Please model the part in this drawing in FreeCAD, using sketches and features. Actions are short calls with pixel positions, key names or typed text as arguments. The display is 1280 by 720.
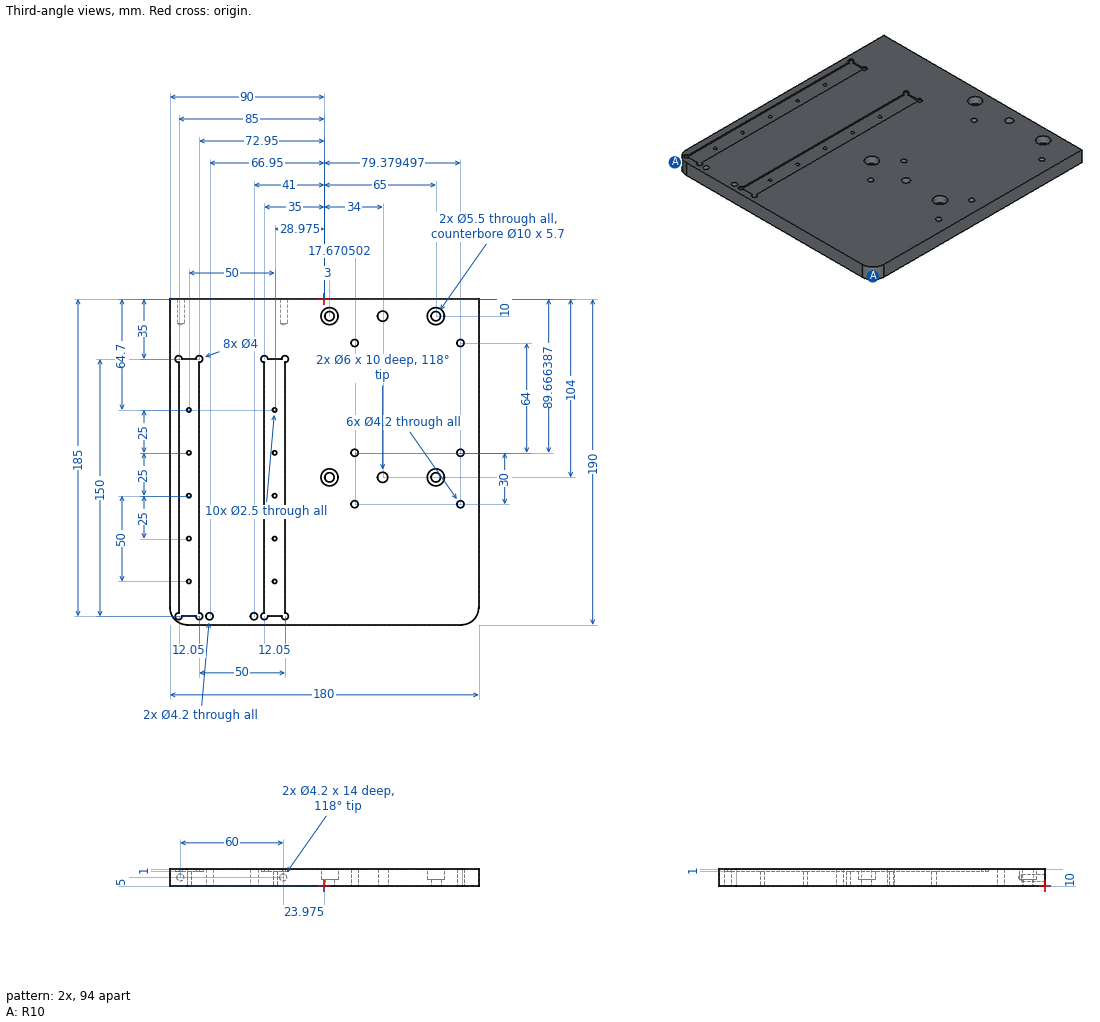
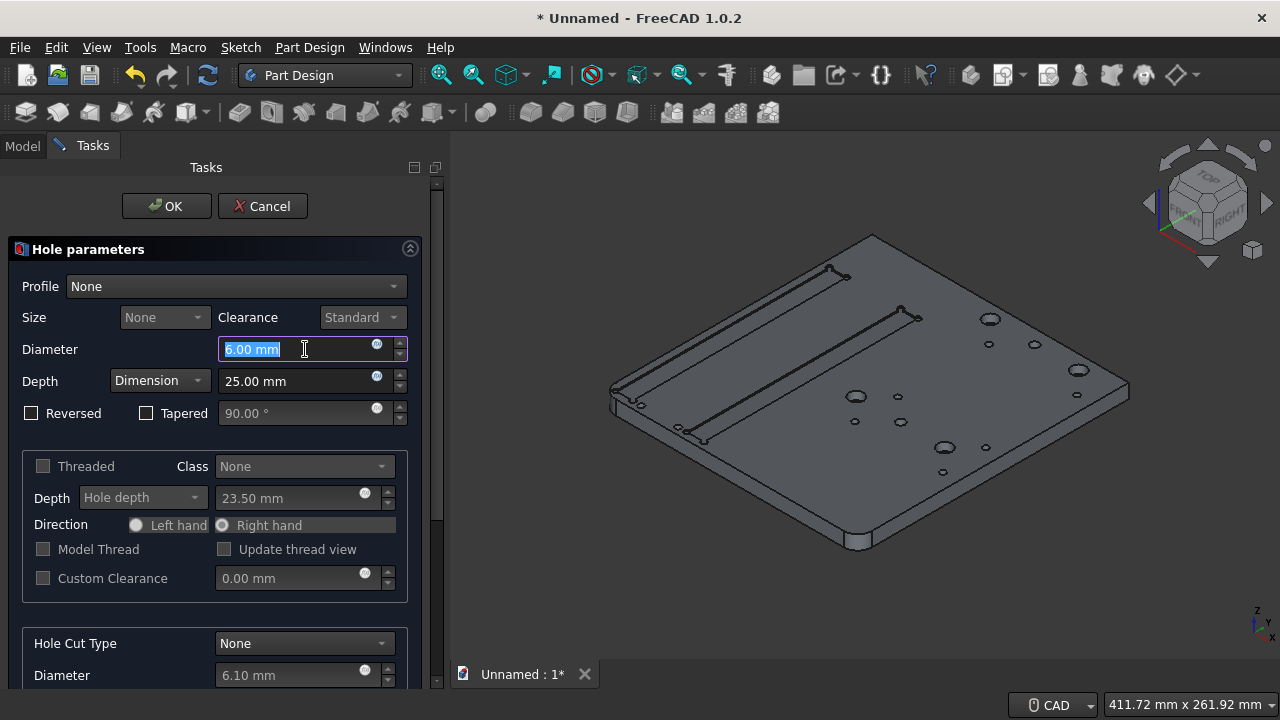
text(6)
key(Tab)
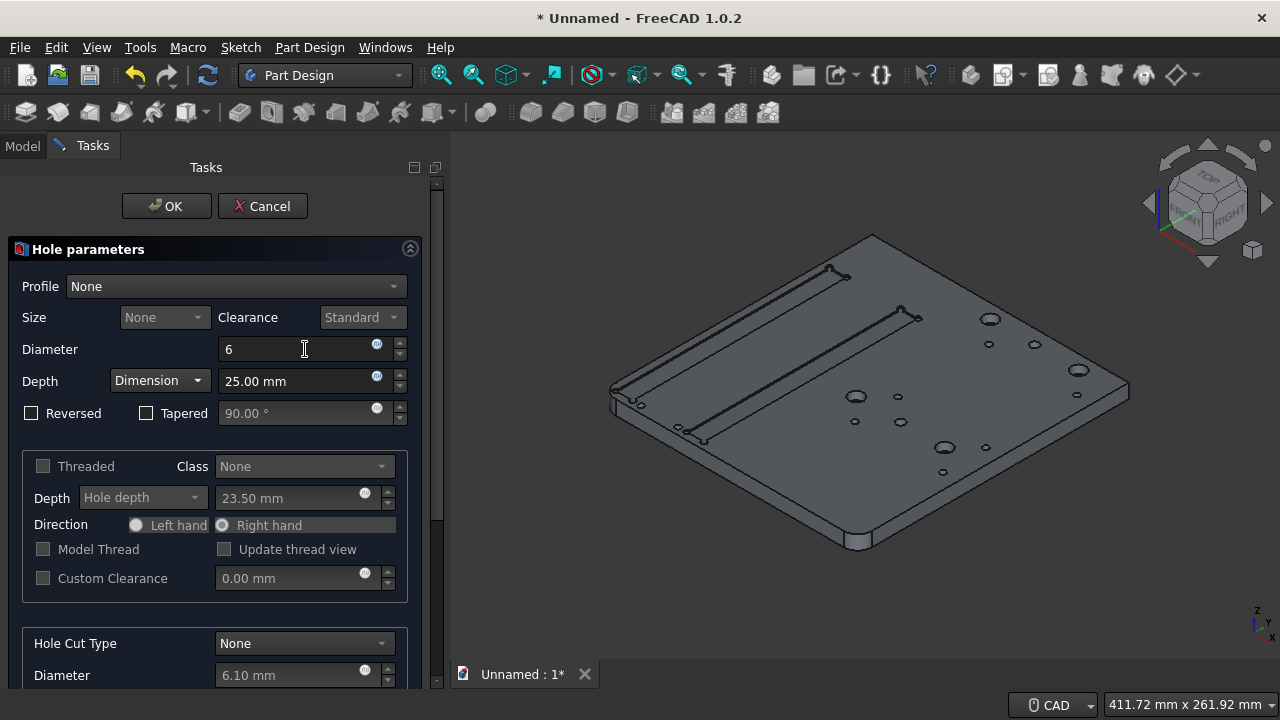
triple_click(305, 381)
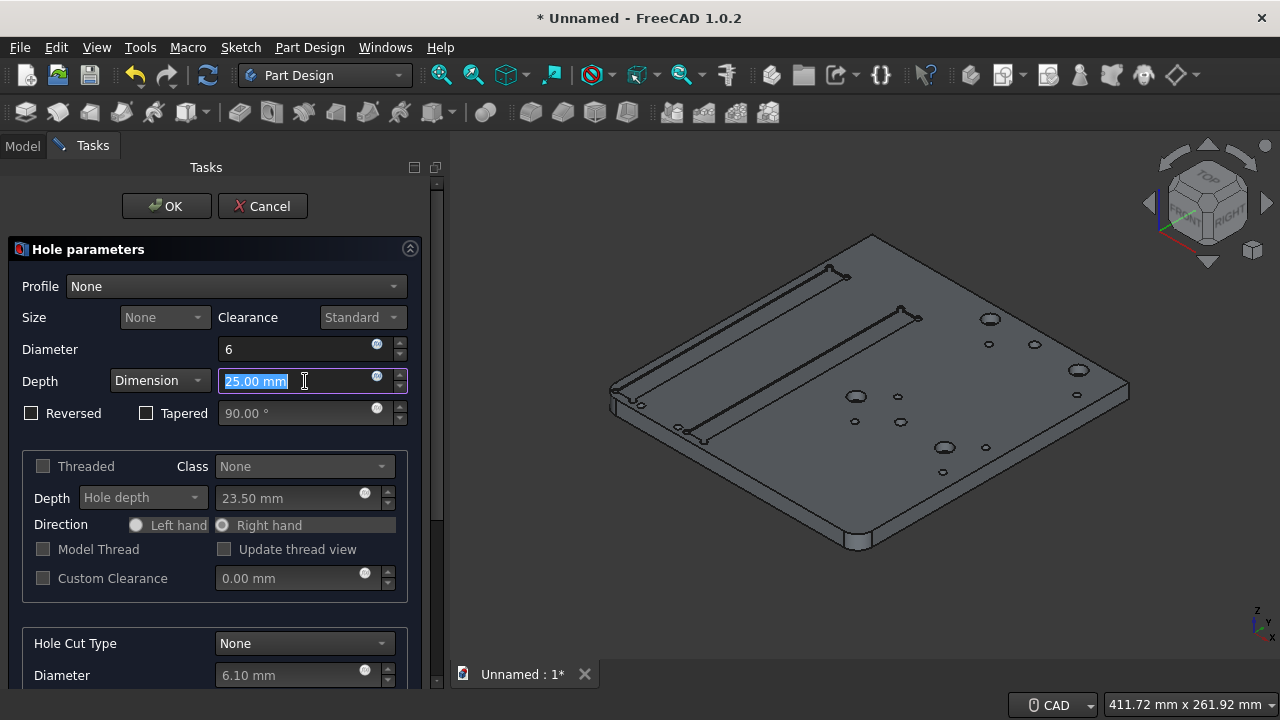
text(10)
key(Tab)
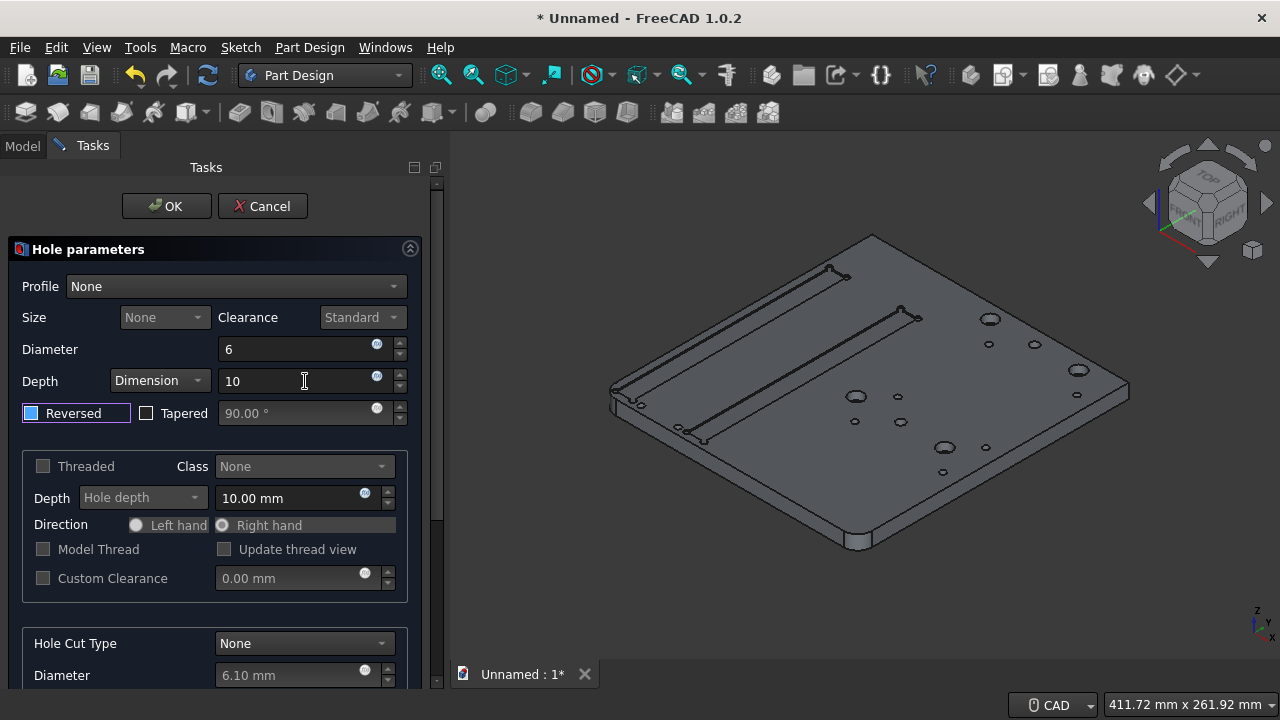
click(167, 206)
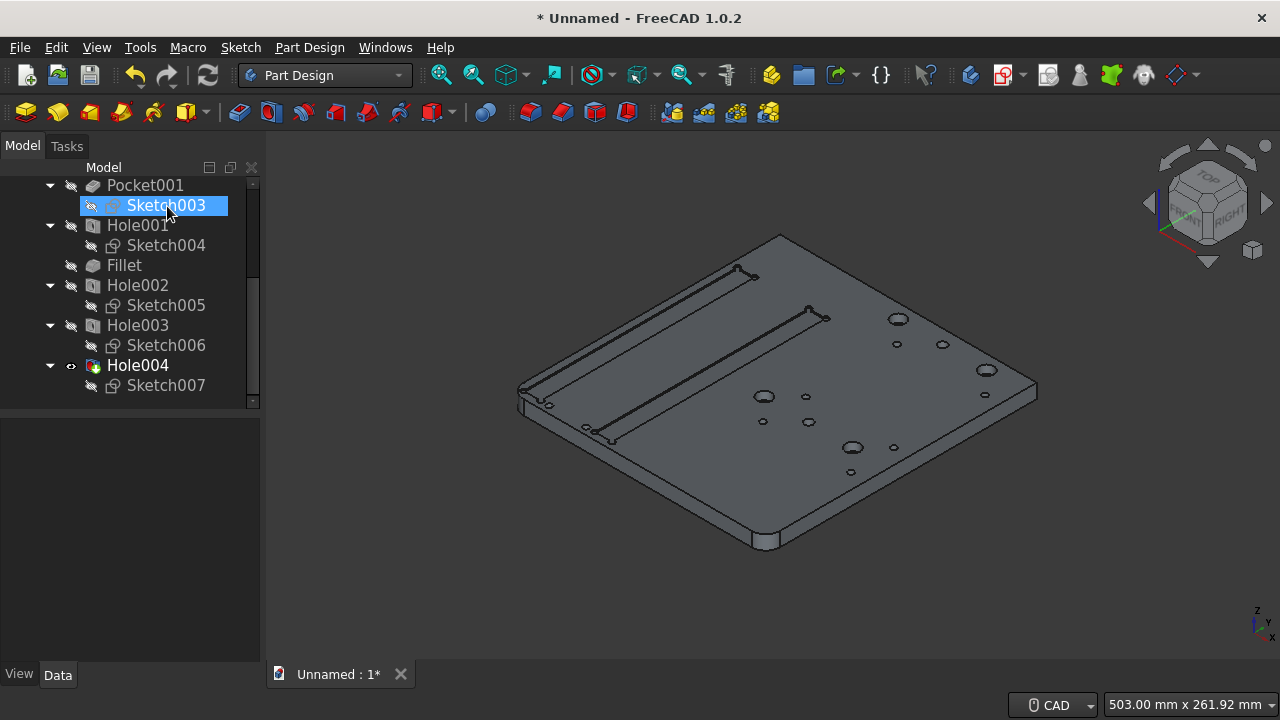
click(769, 473)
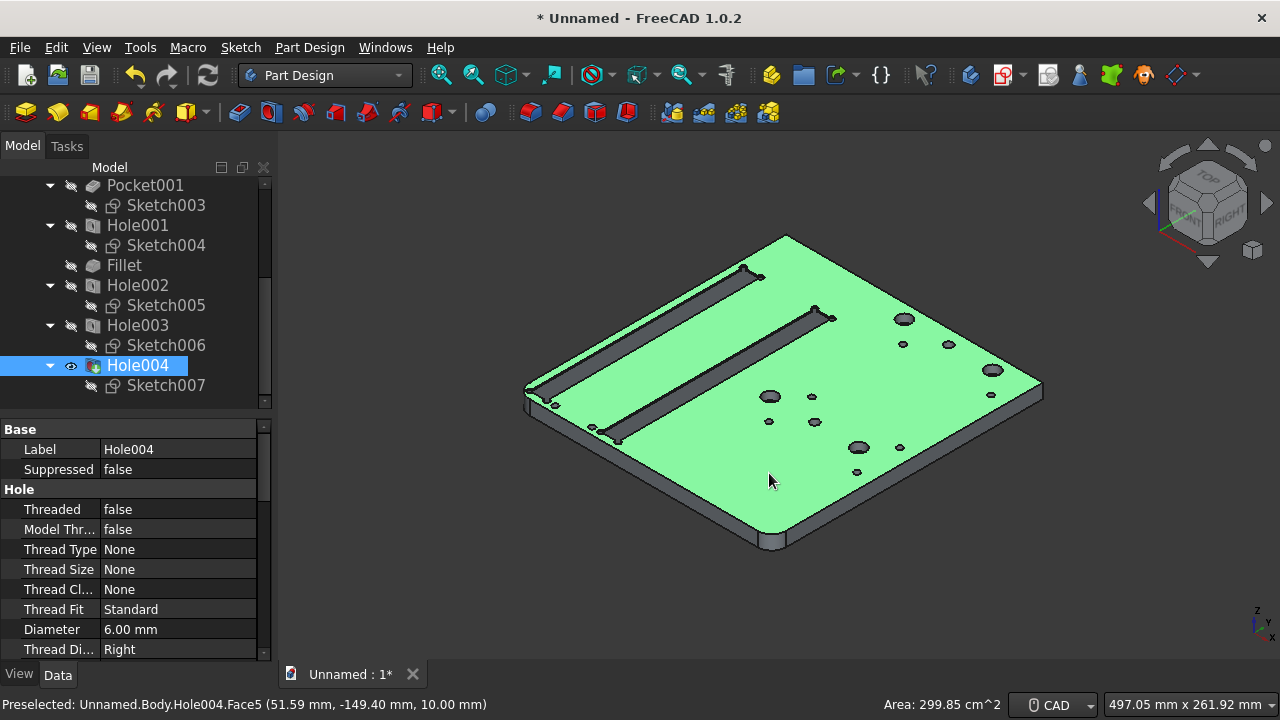
click(1004, 76)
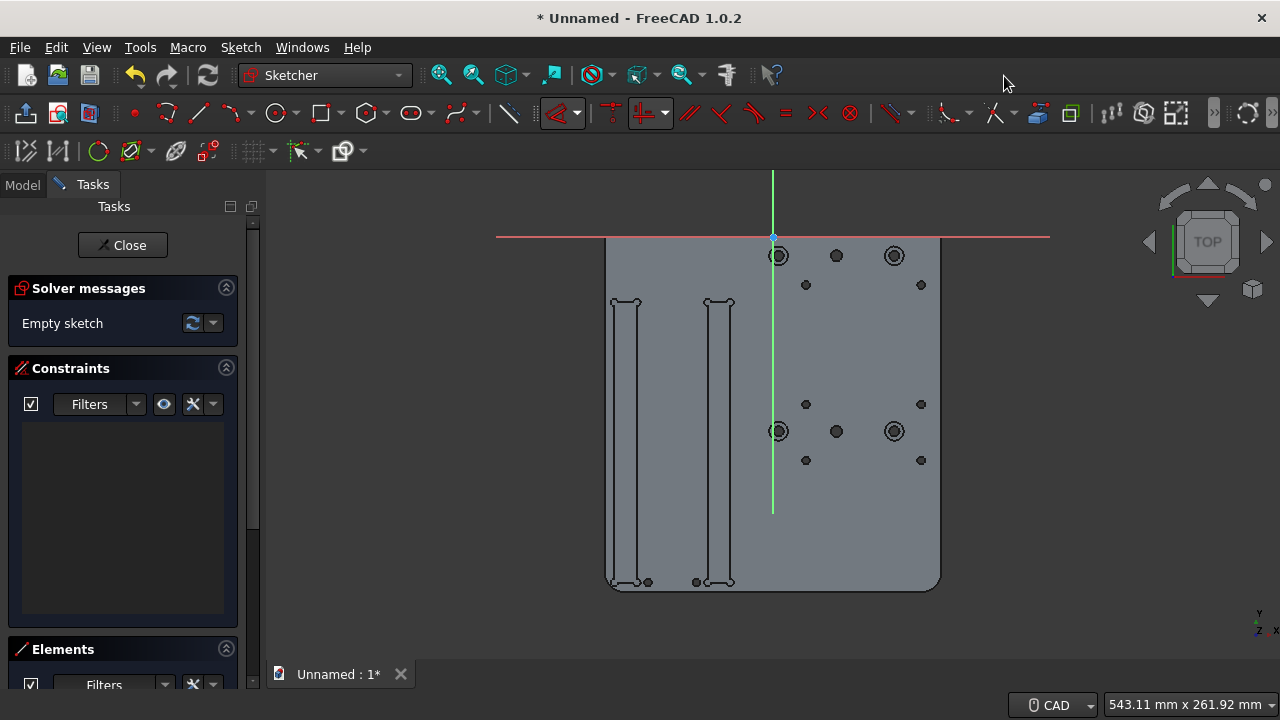
key(g)
key(c)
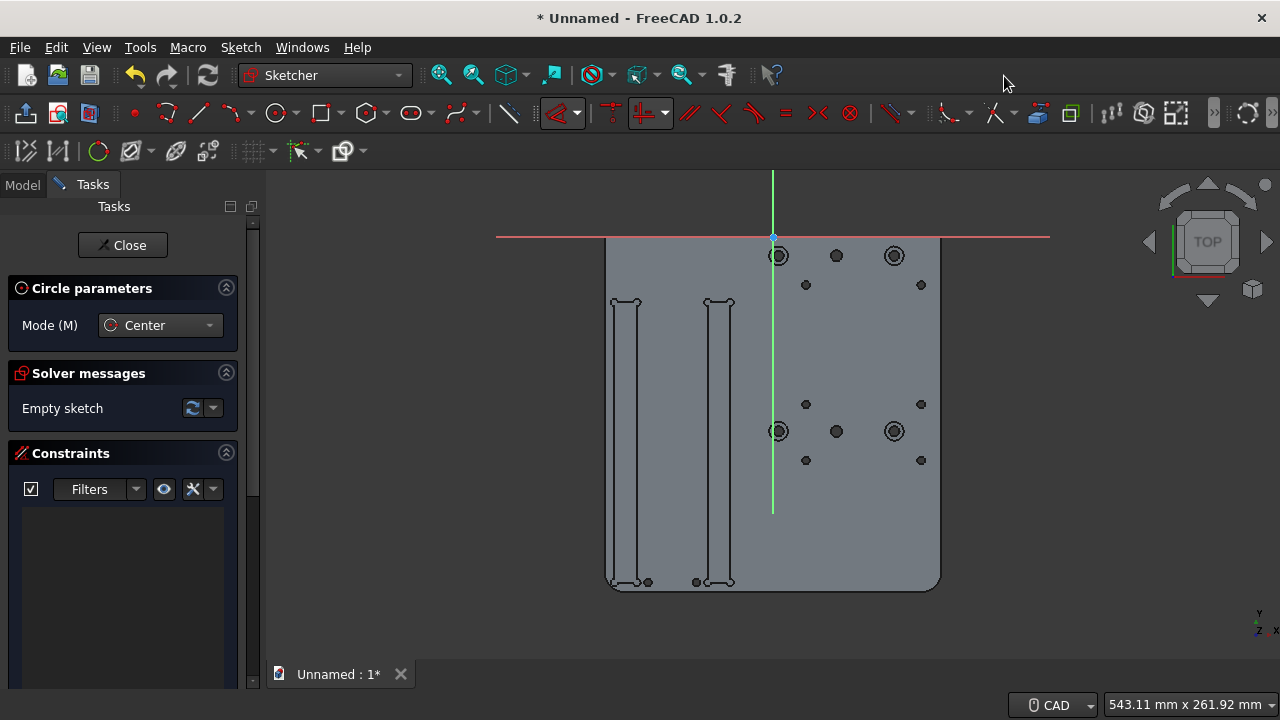
scroll(719, 358, up, 12)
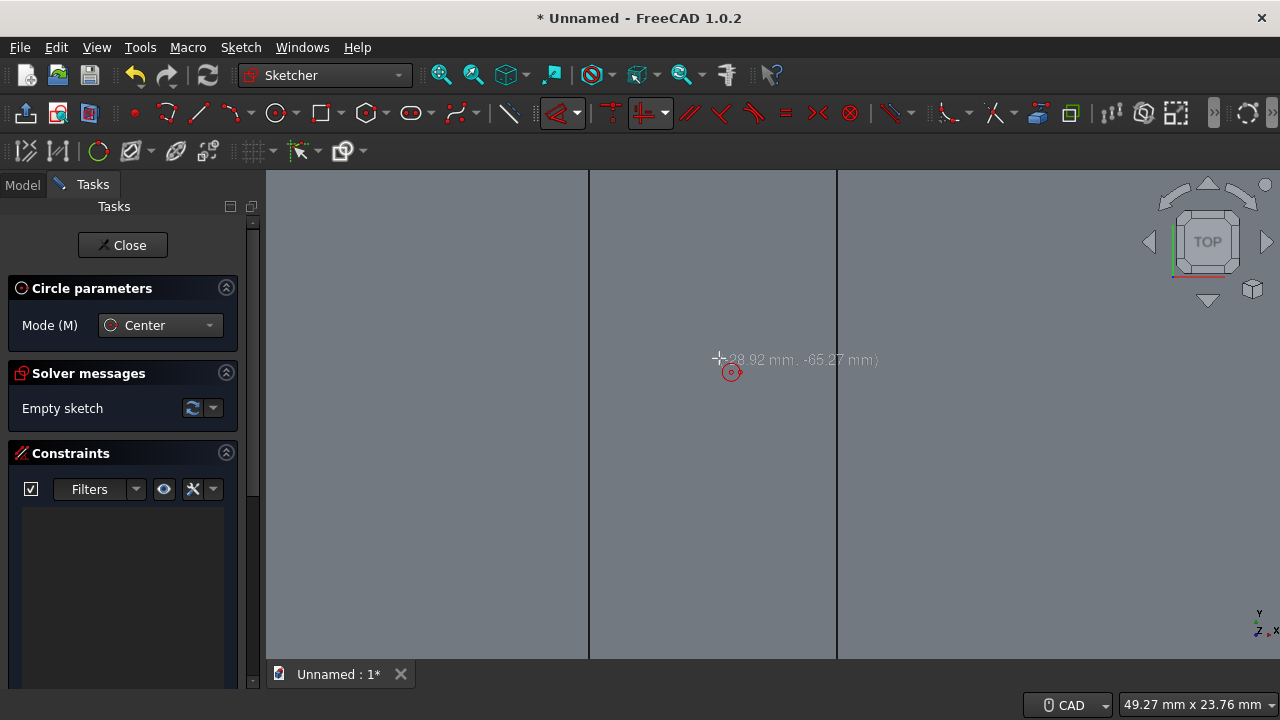
scroll(726, 383, down, 12)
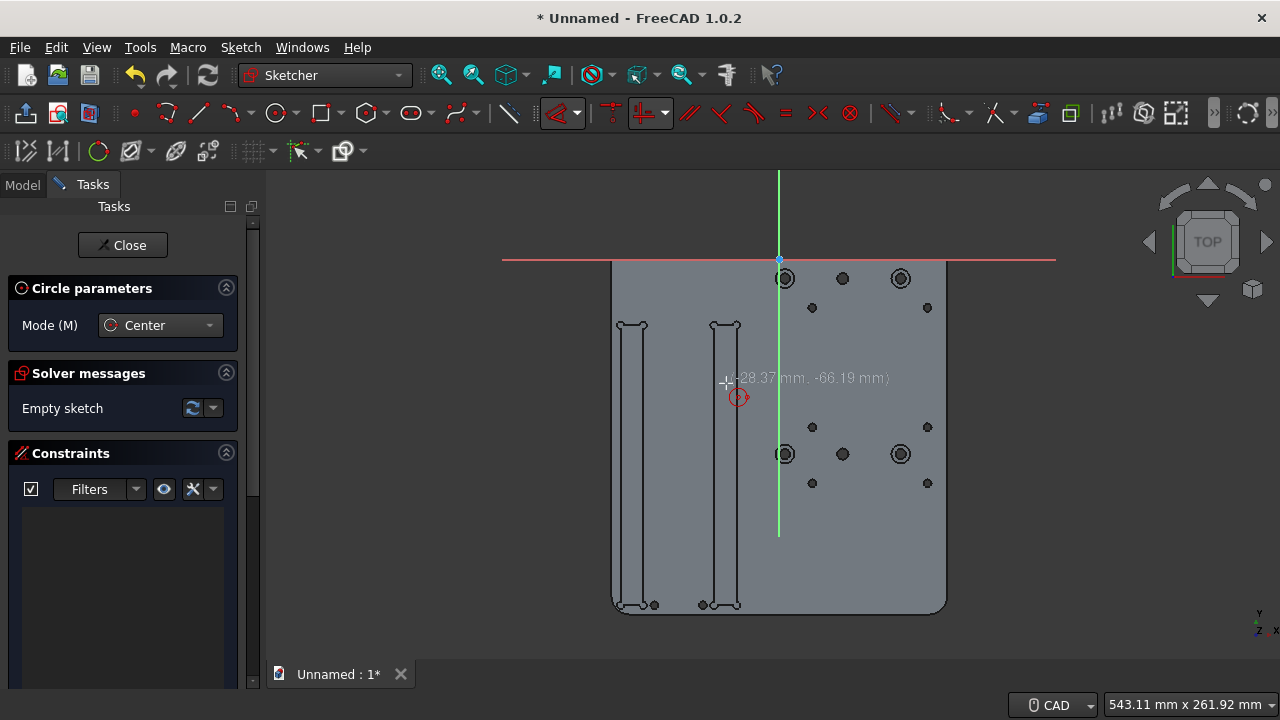
click(725, 381)
move(727, 379)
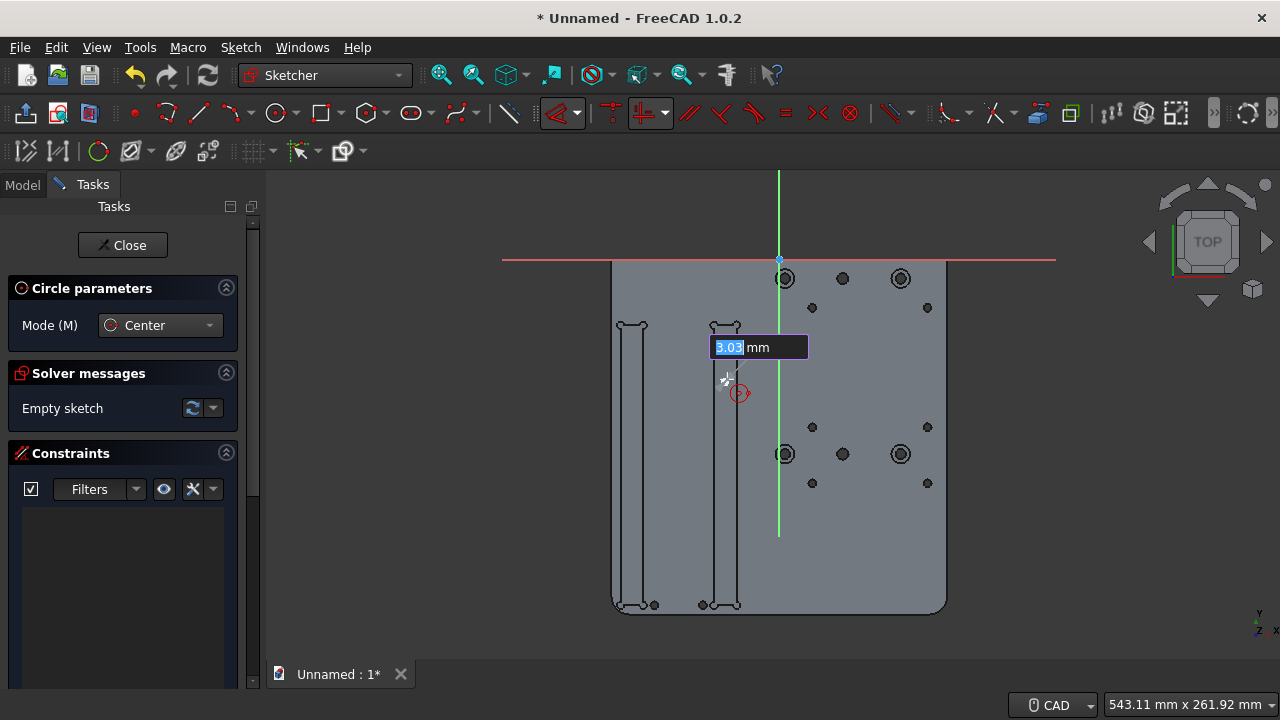
text(2.5)
key(Return)